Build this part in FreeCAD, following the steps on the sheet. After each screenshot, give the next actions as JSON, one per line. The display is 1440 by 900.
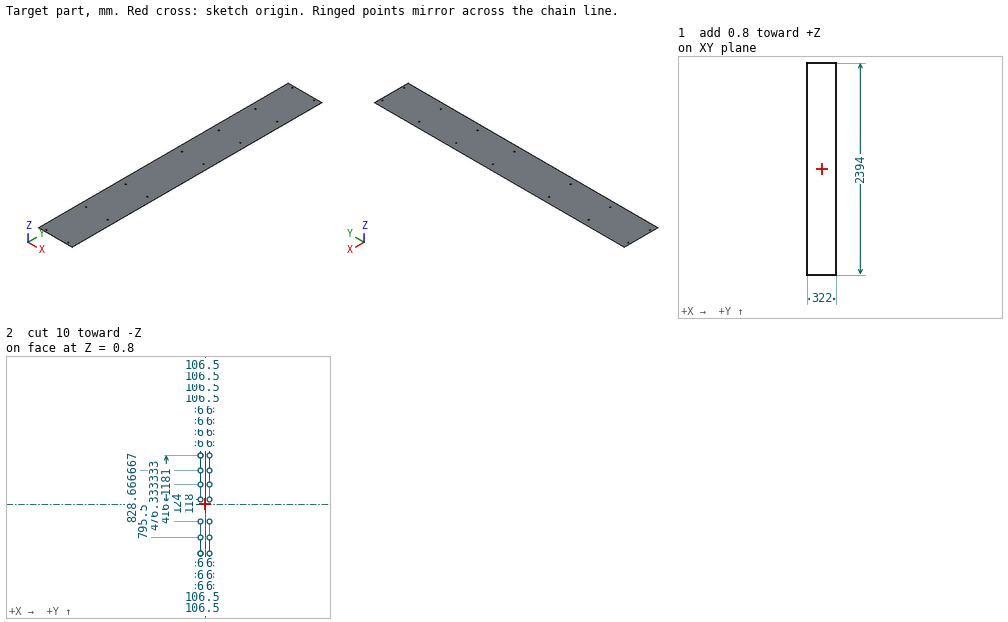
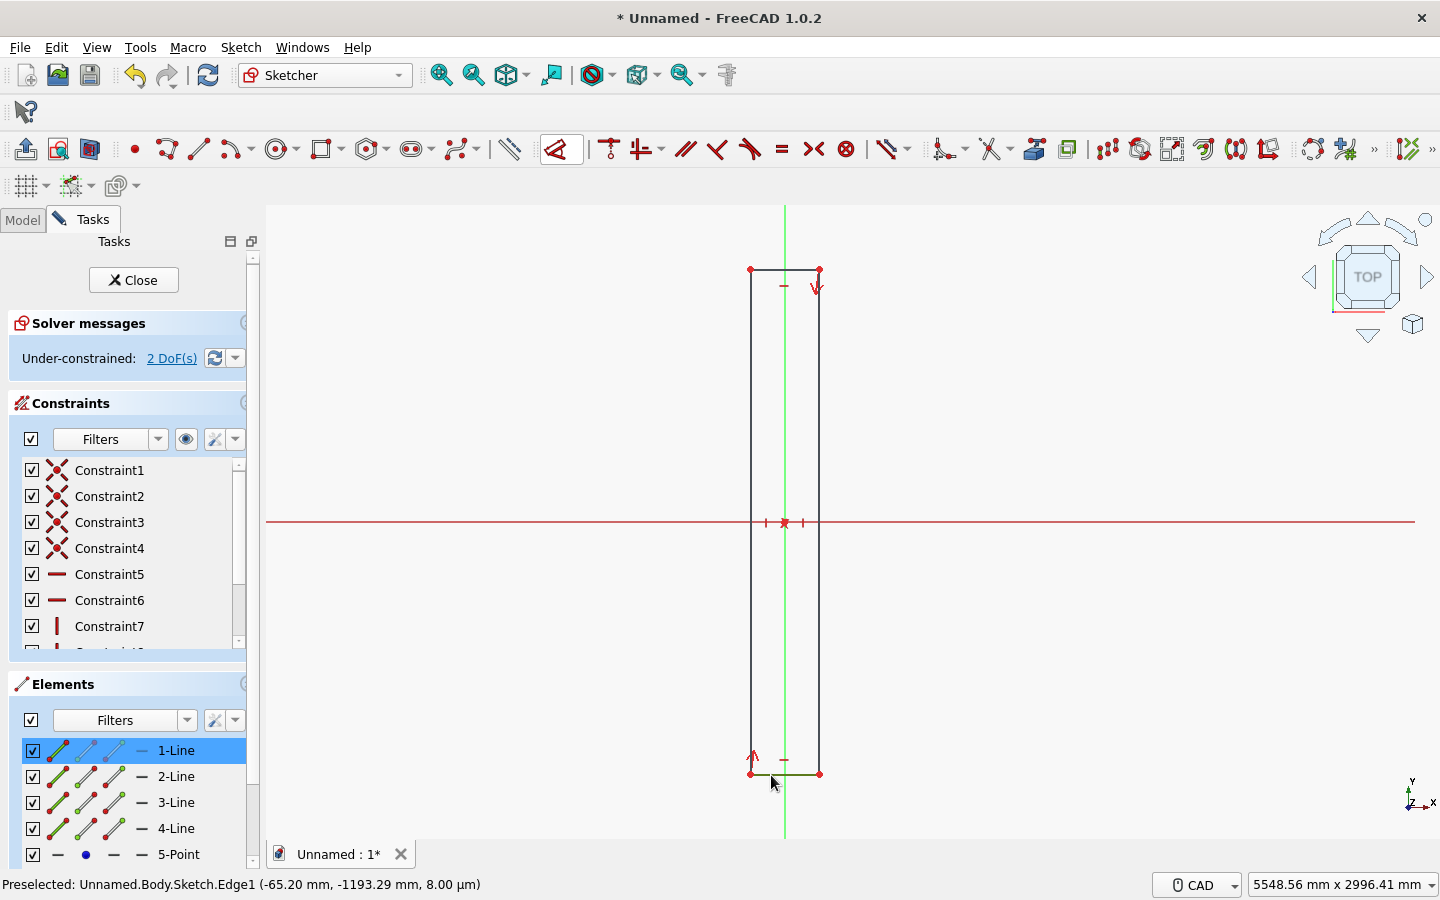
{"action": "key", "text": "l"}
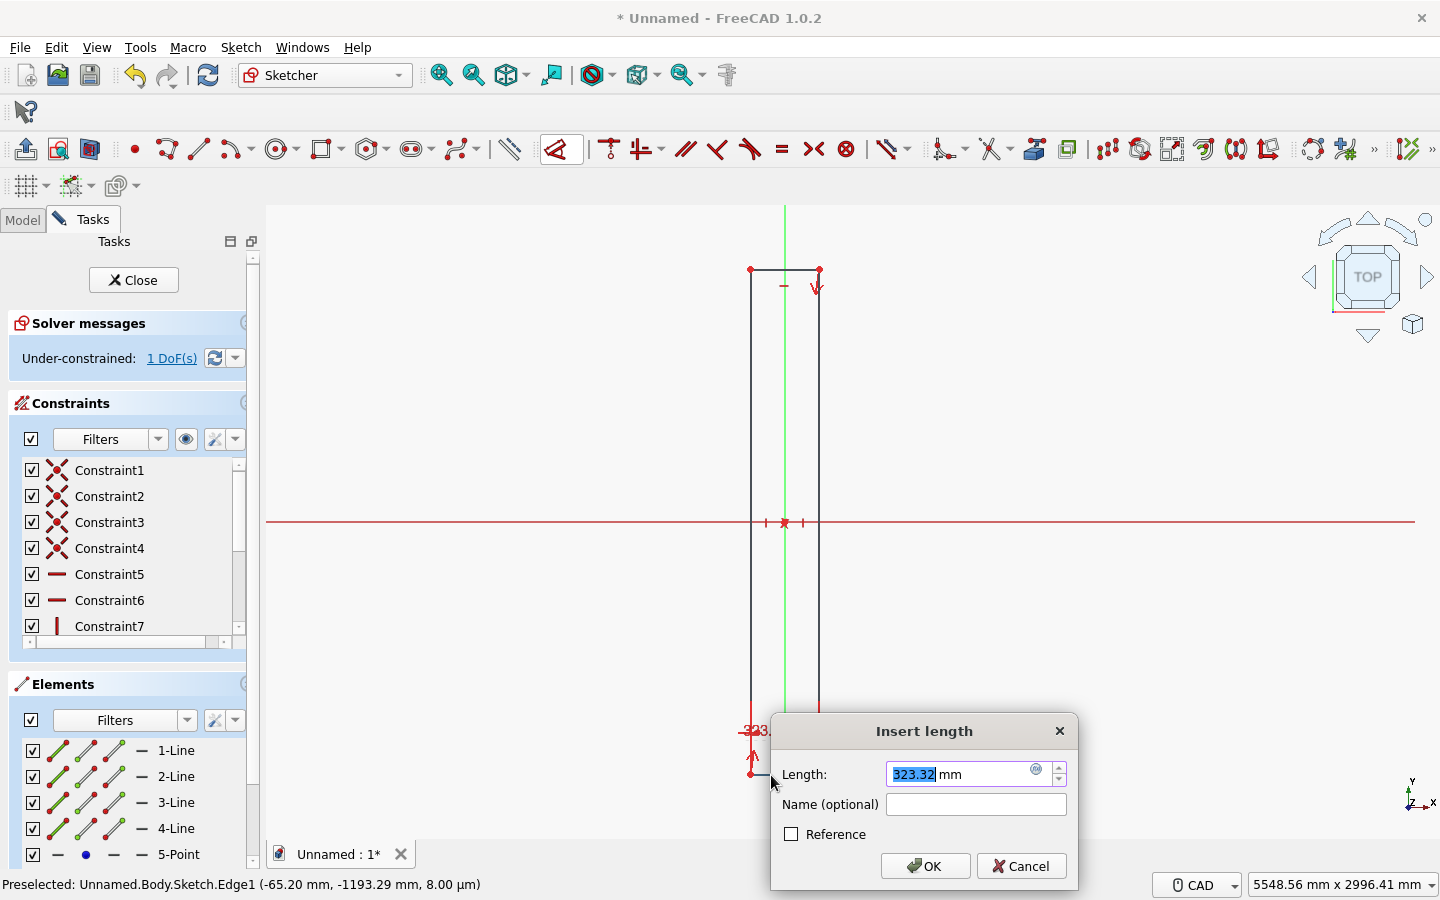
{"action": "type", "text": "322"}
{"action": "key", "text": "Return"}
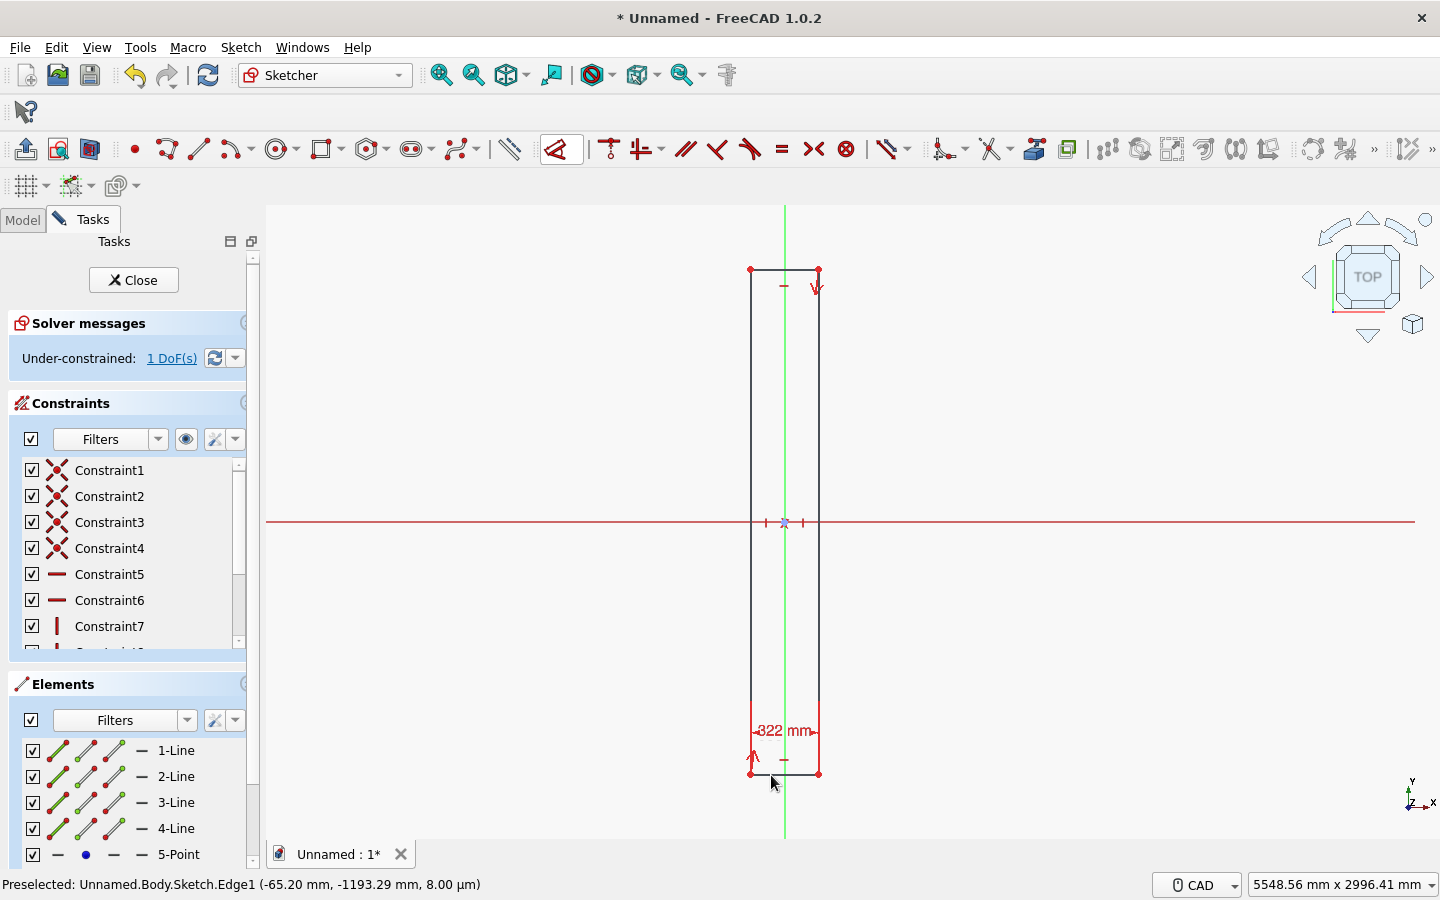
{"action": "left_click", "coordinate": [819, 623]}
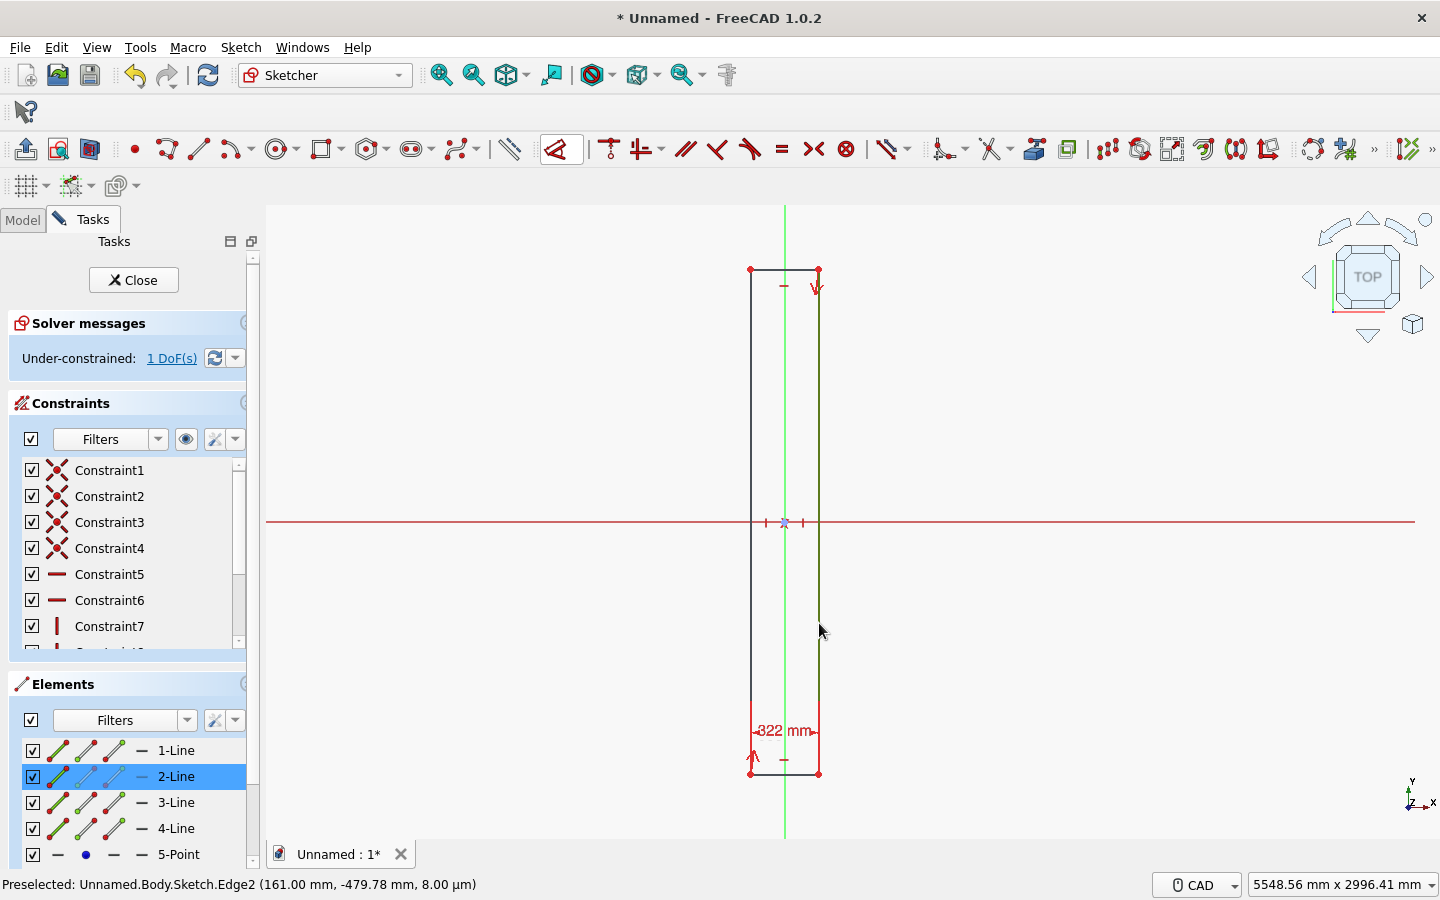
{"action": "left_click", "coordinate": [578, 150]}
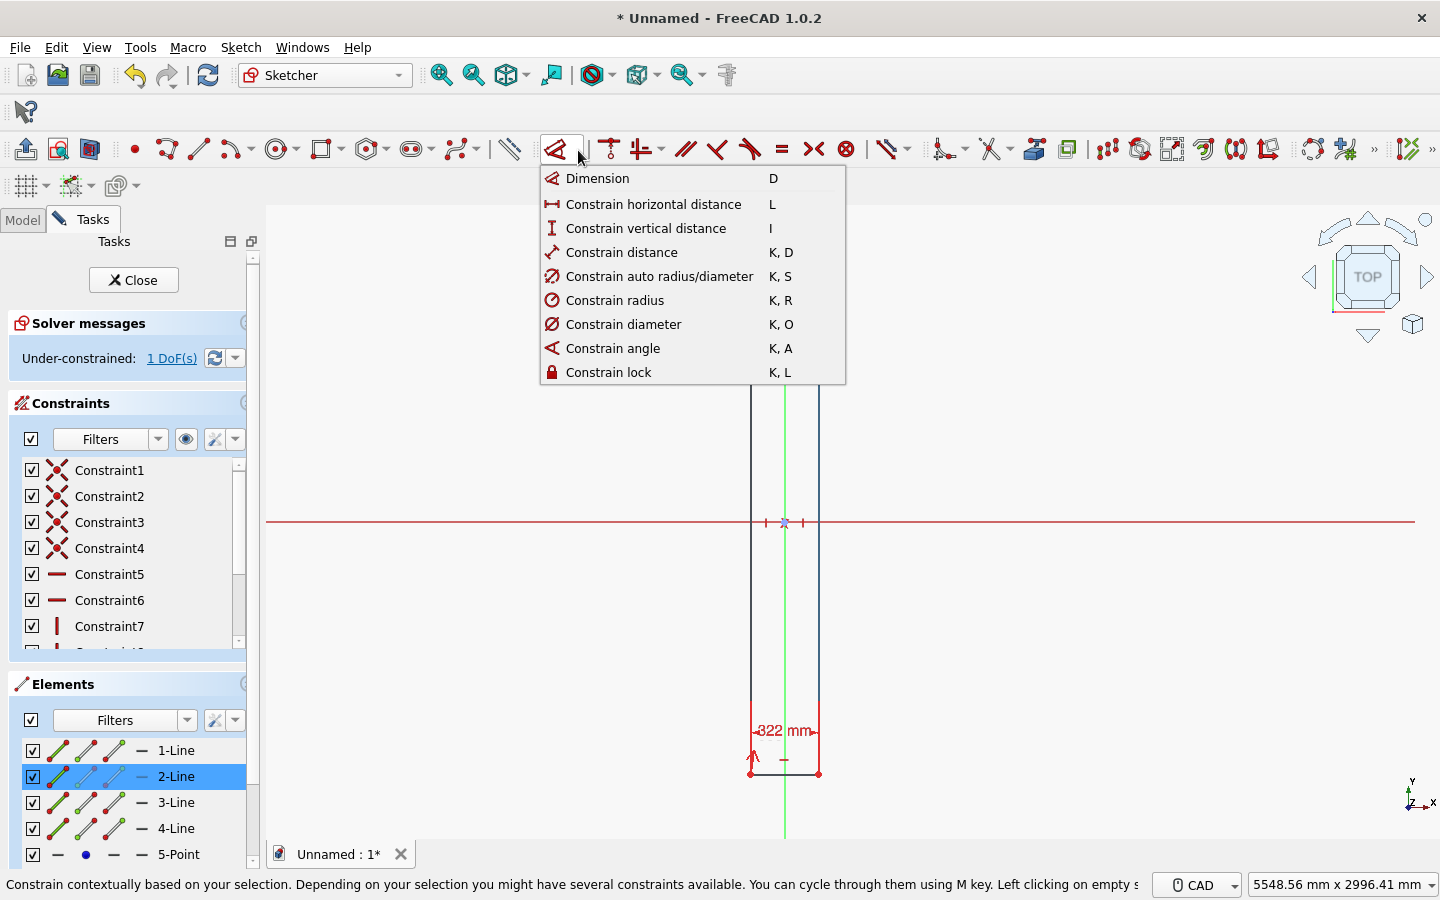
{"action": "left_click", "coordinate": [693, 228]}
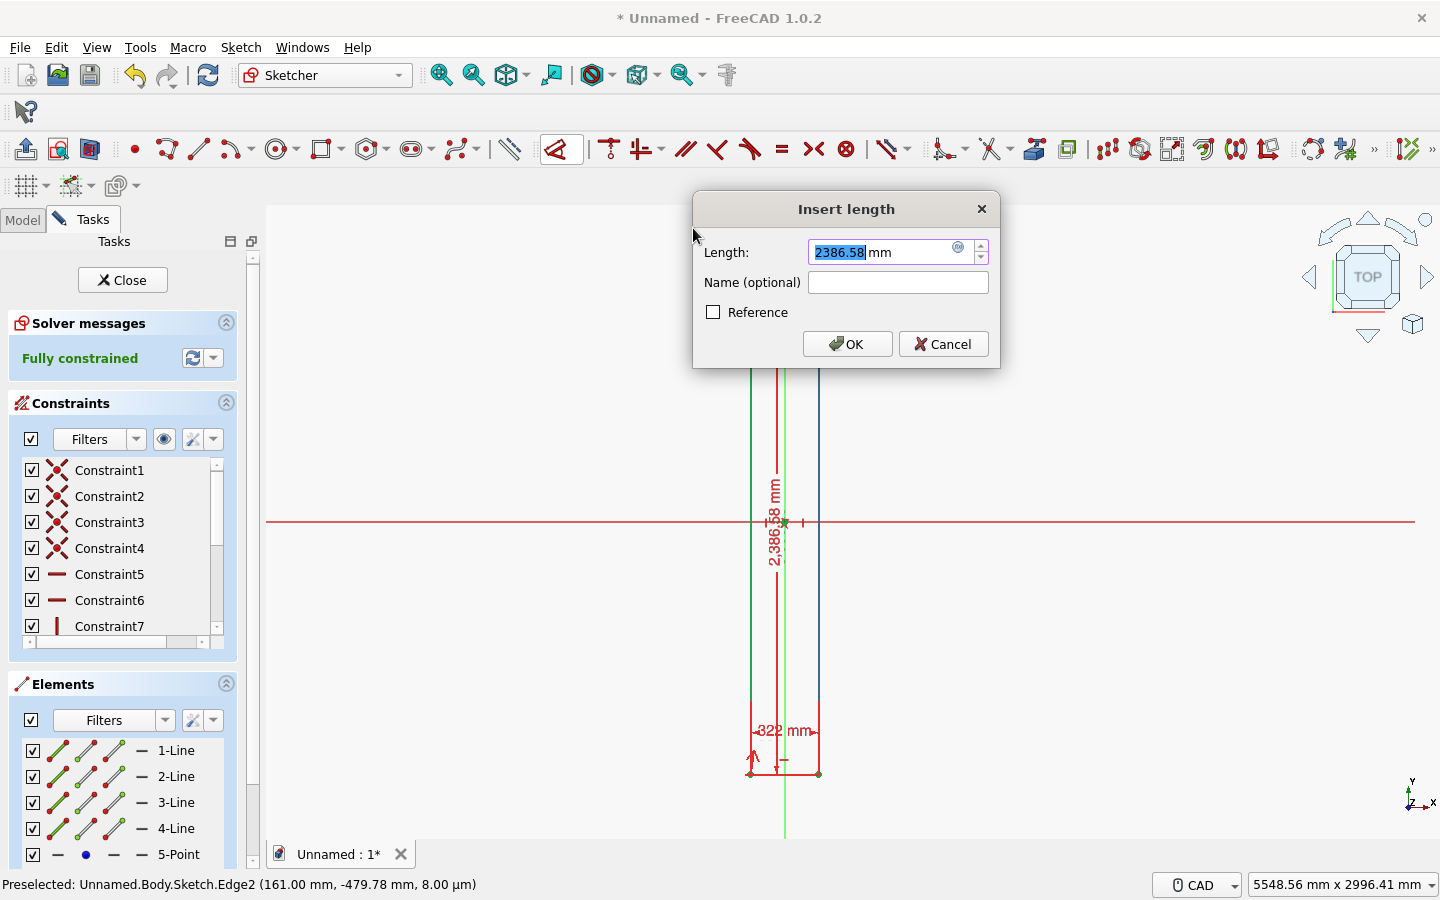
{"action": "type", "text": "2394"}
{"action": "key", "text": "Return"}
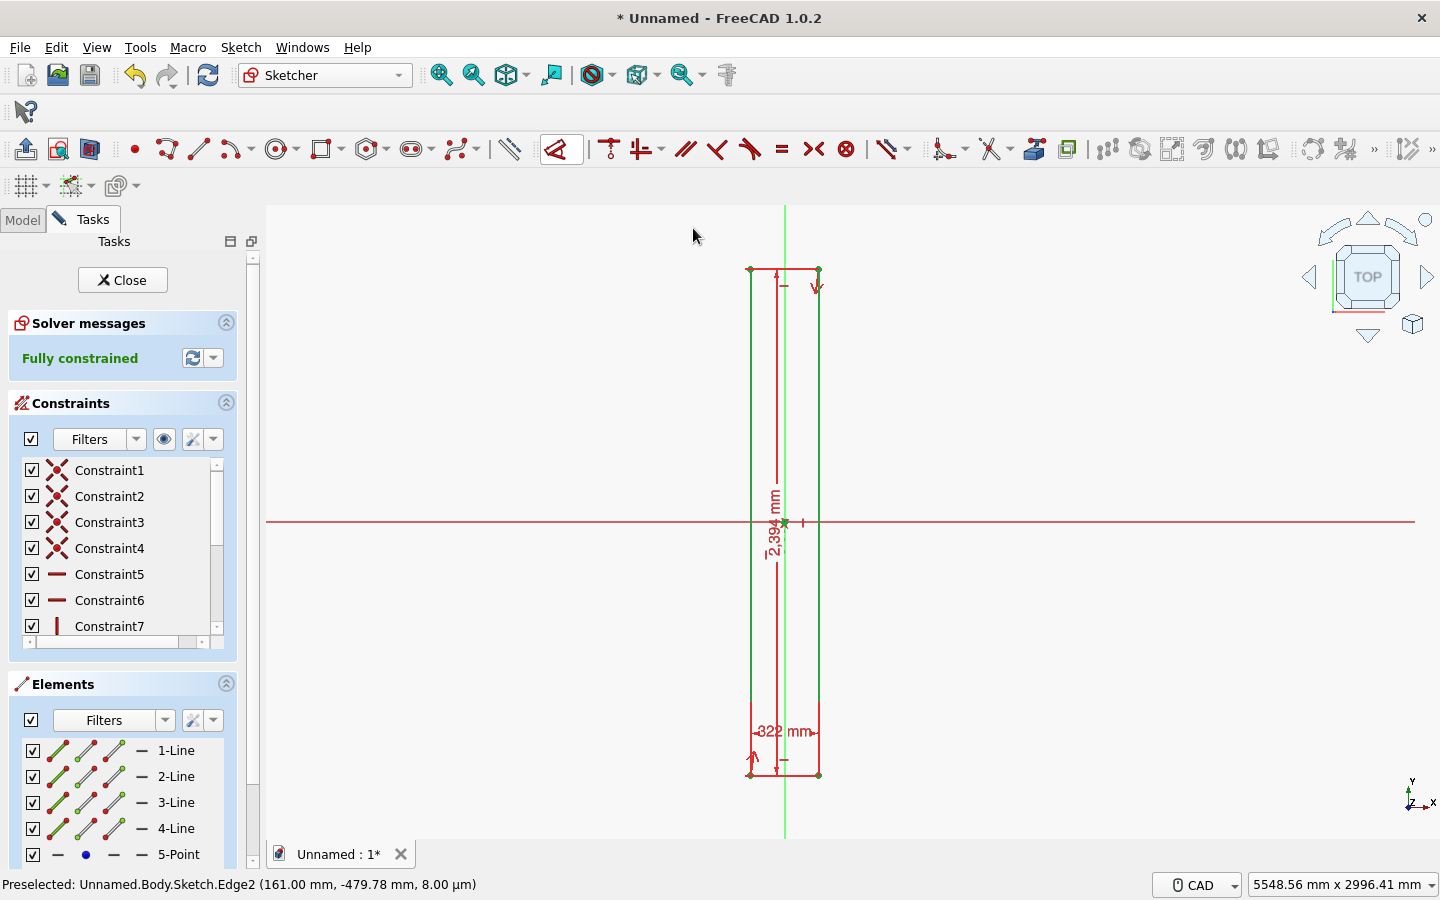
{"action": "left_click", "coordinate": [123, 280]}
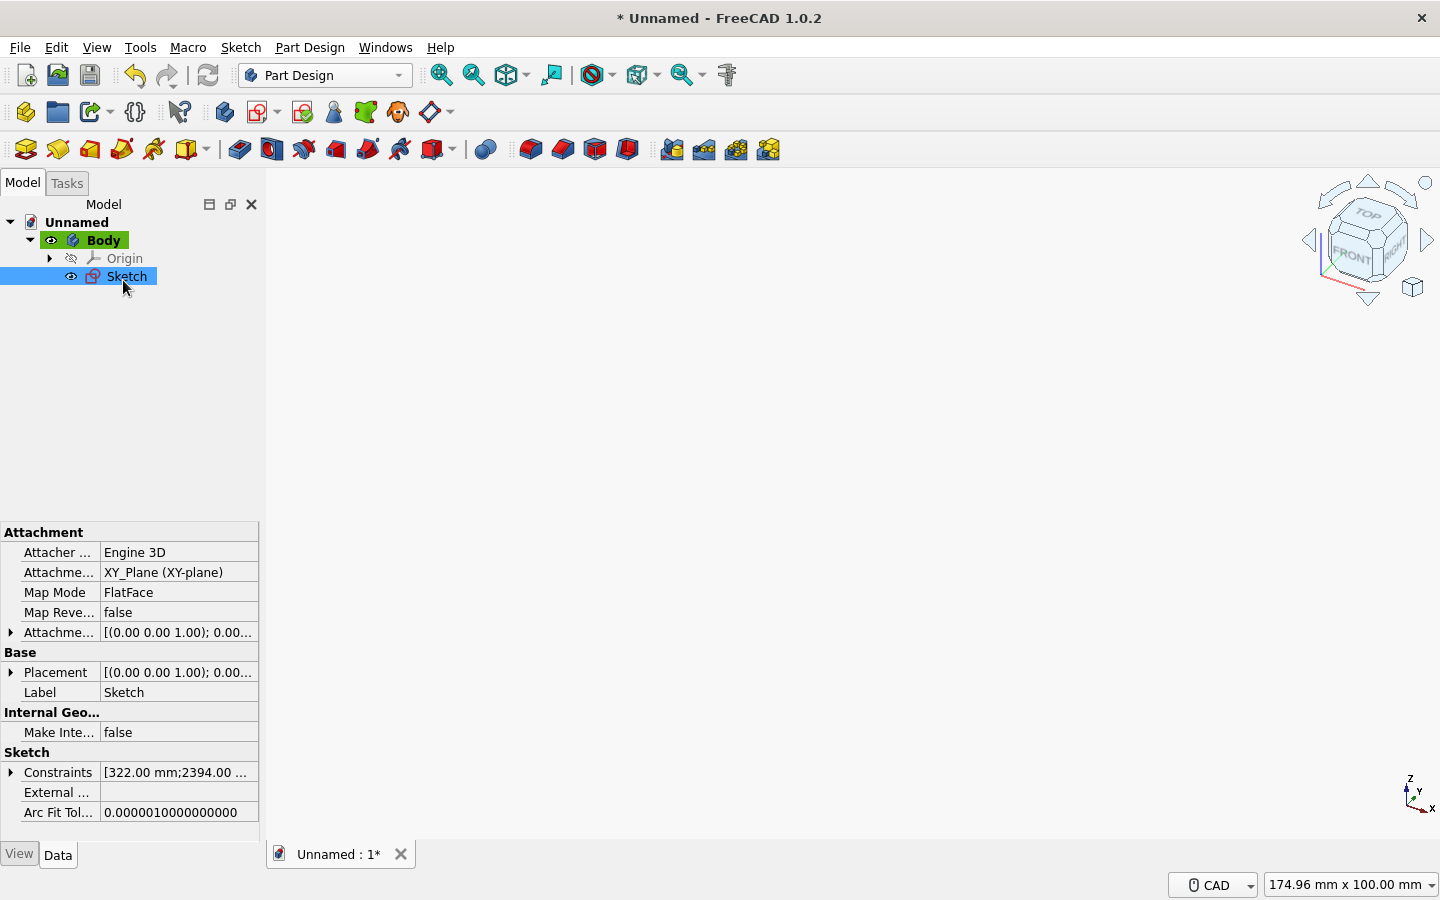
{"action": "left_click", "coordinate": [26, 150]}